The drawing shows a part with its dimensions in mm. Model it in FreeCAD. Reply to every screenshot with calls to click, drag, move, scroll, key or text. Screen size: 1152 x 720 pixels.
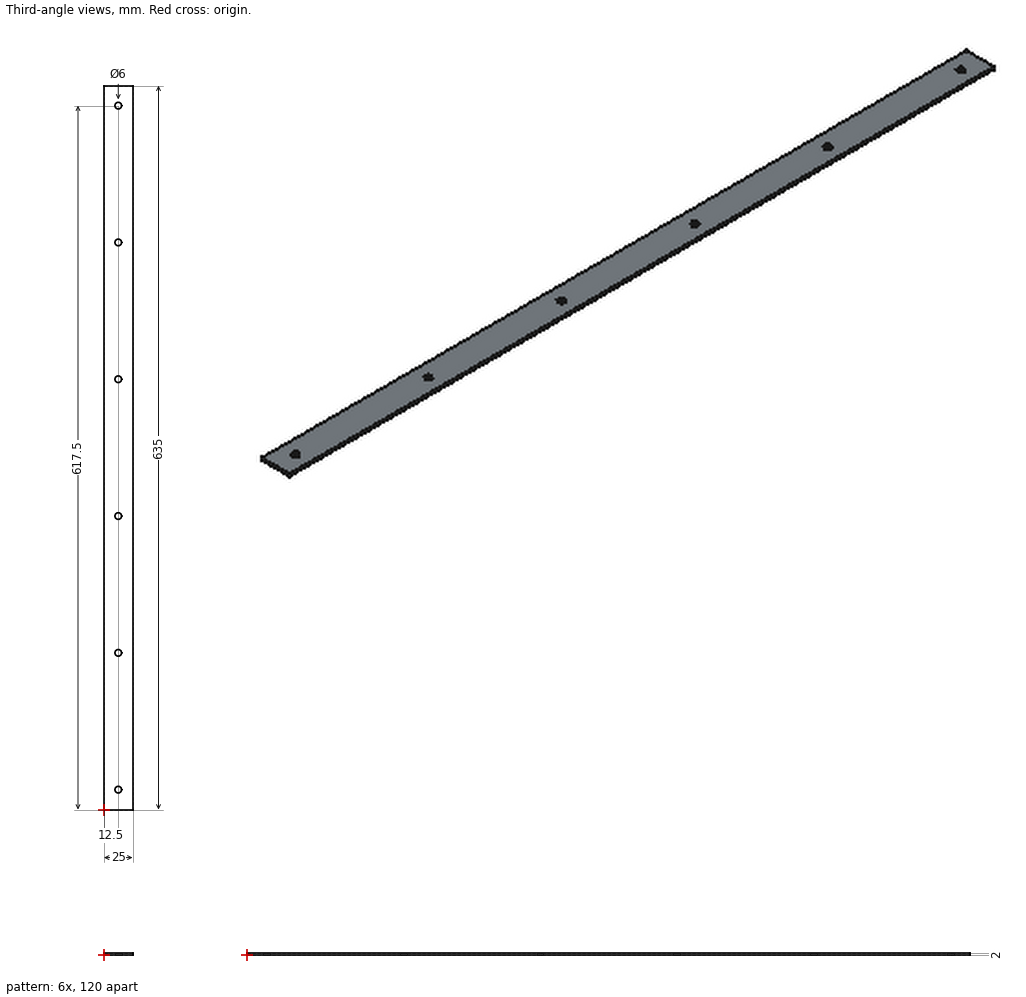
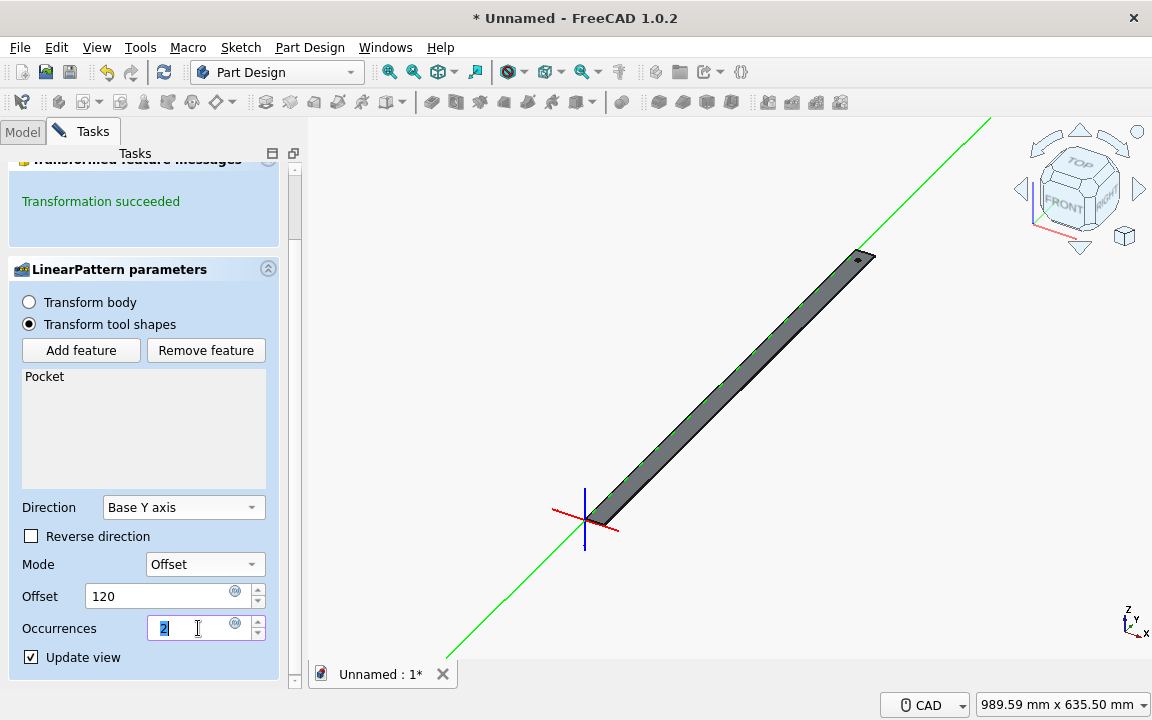
text(6)
key(Tab)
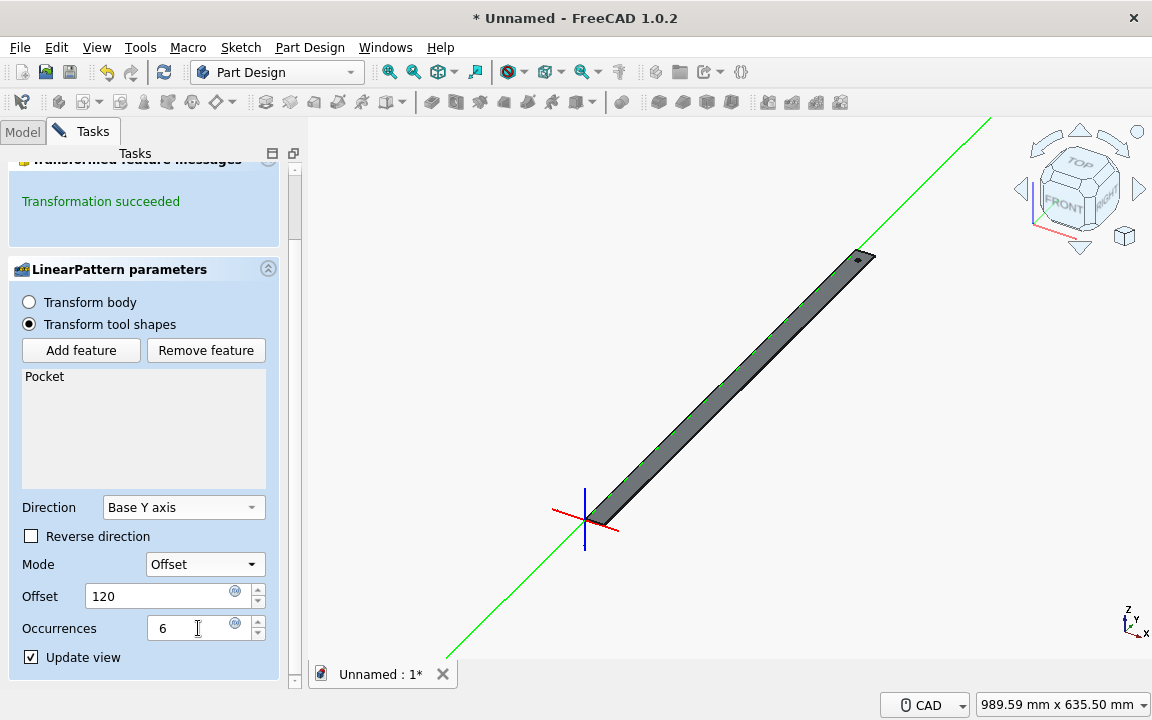
click(30, 536)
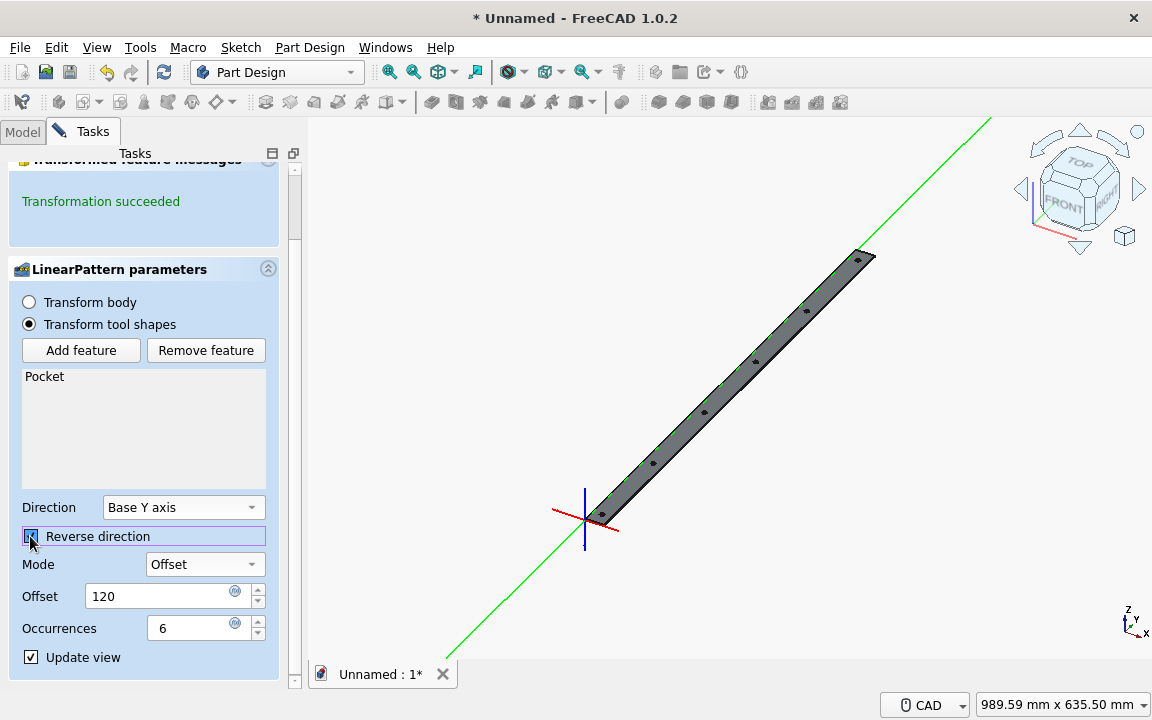
scroll(295, 426, up, 3)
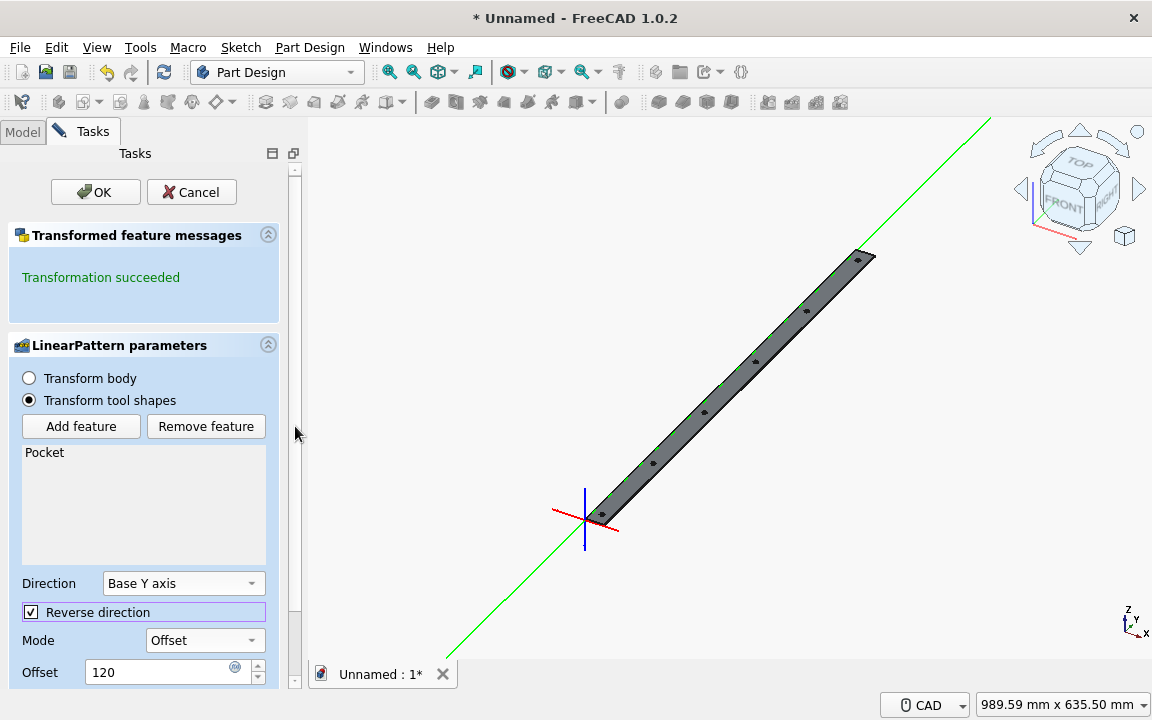
click(96, 192)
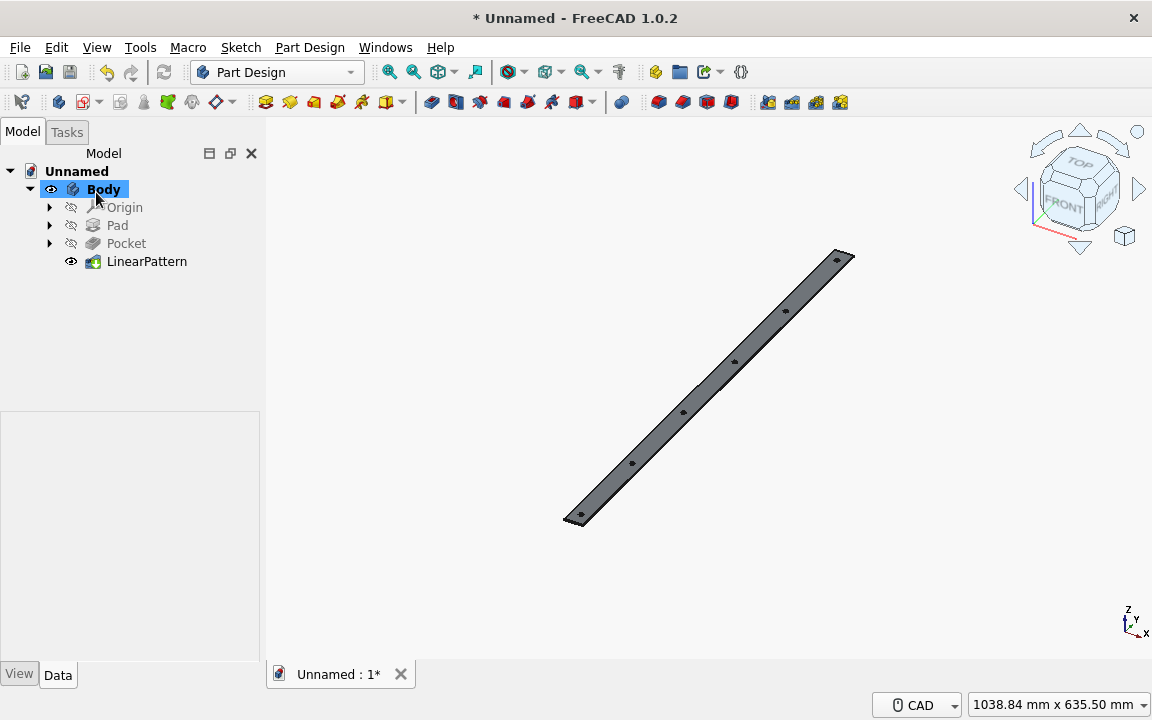
key(0)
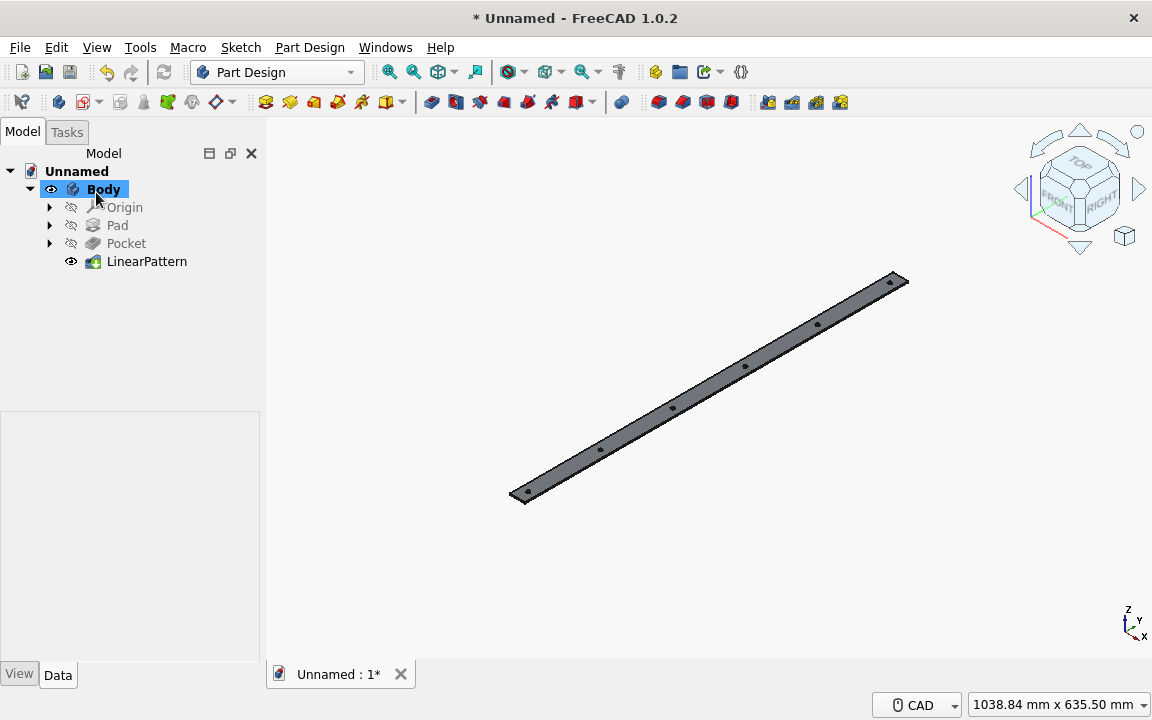
click(390, 72)